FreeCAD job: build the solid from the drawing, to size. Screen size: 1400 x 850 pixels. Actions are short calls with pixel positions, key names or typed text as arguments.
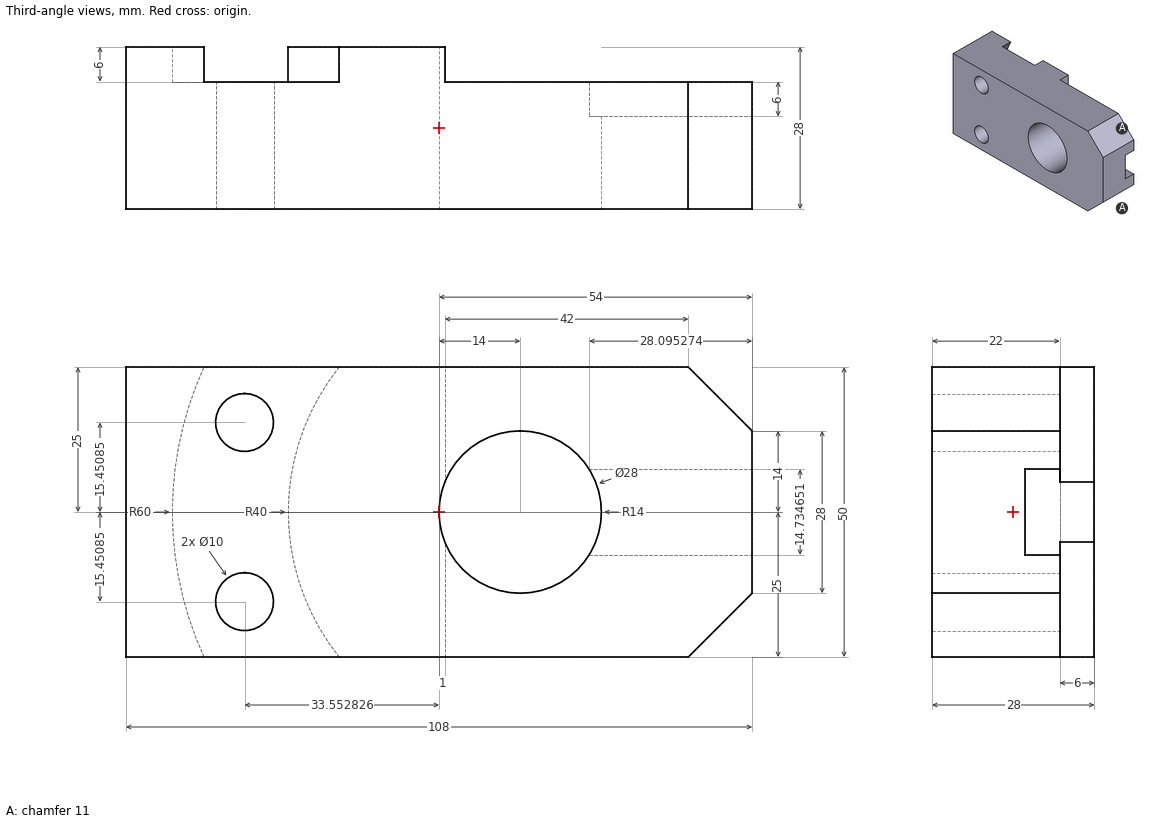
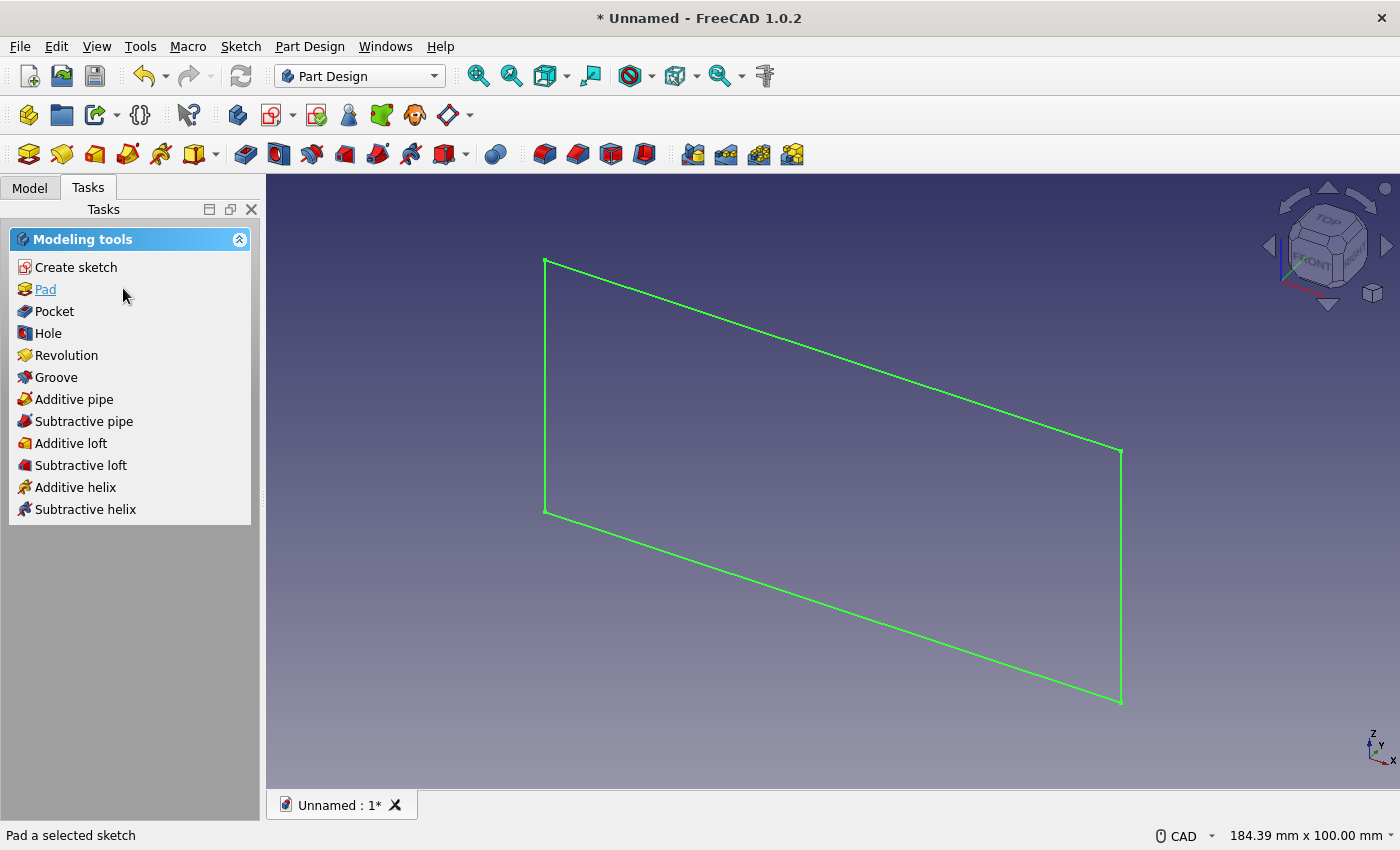
click(29, 154)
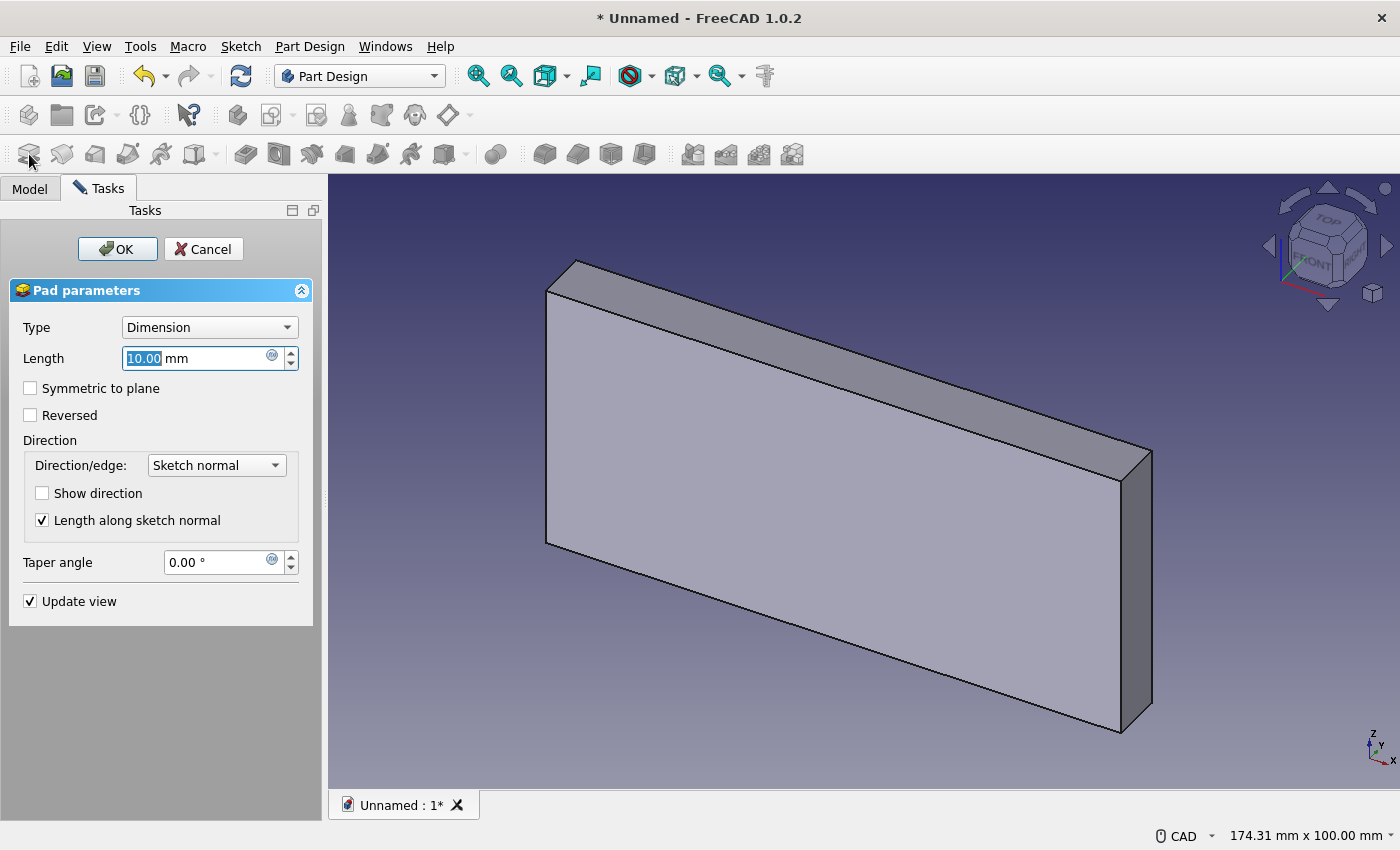
text(28)
key(Tab)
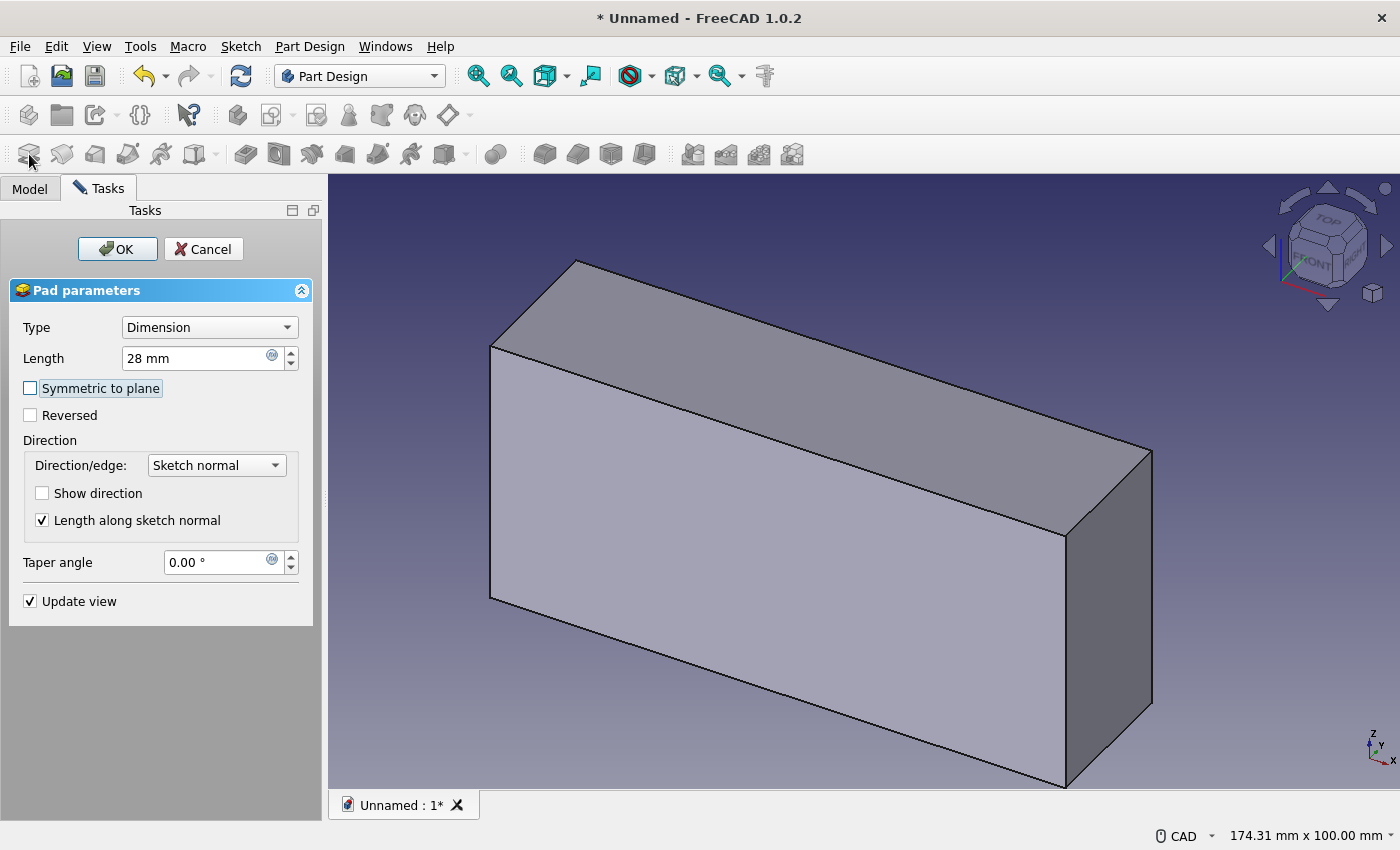
click(31, 388)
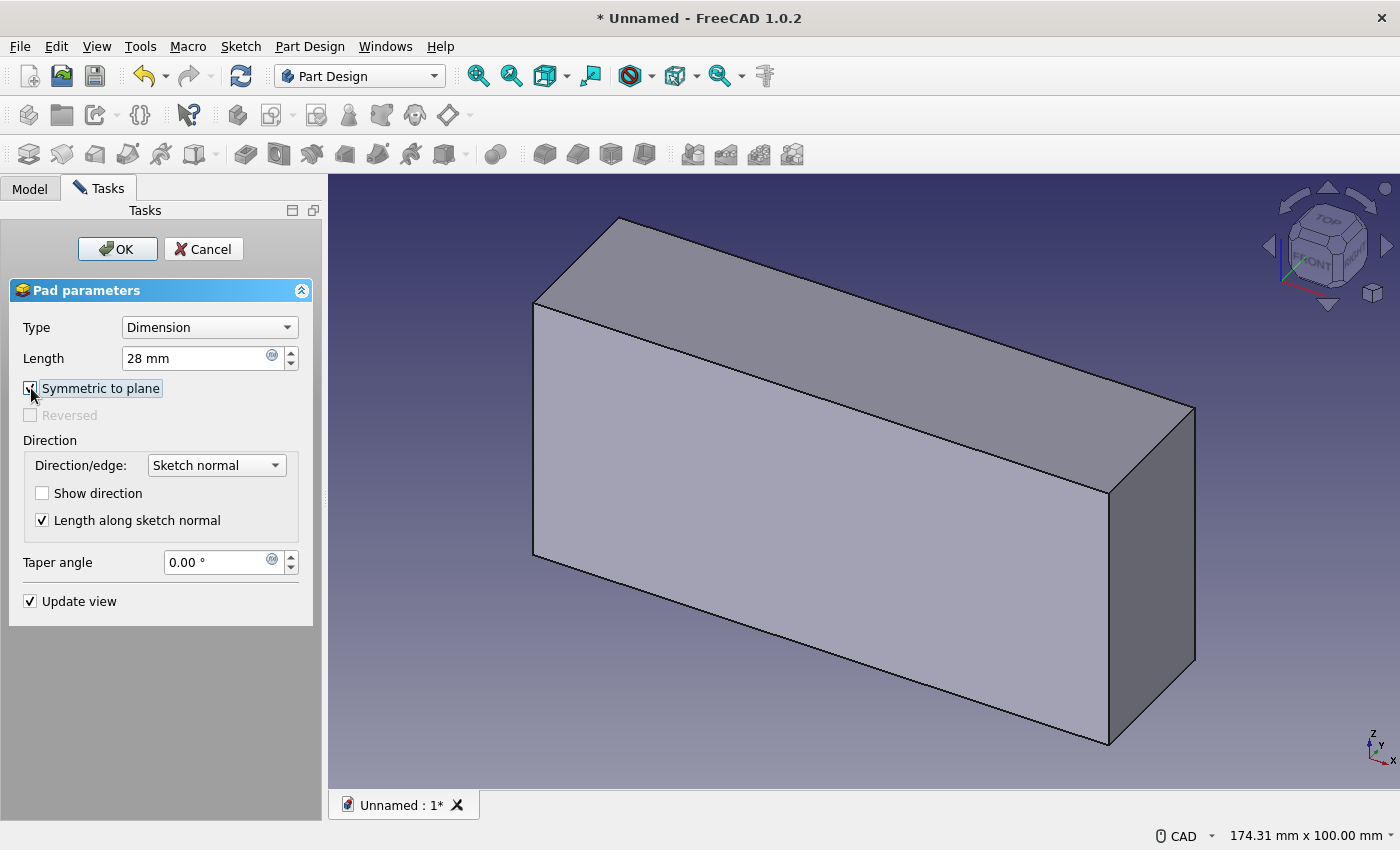
click(118, 249)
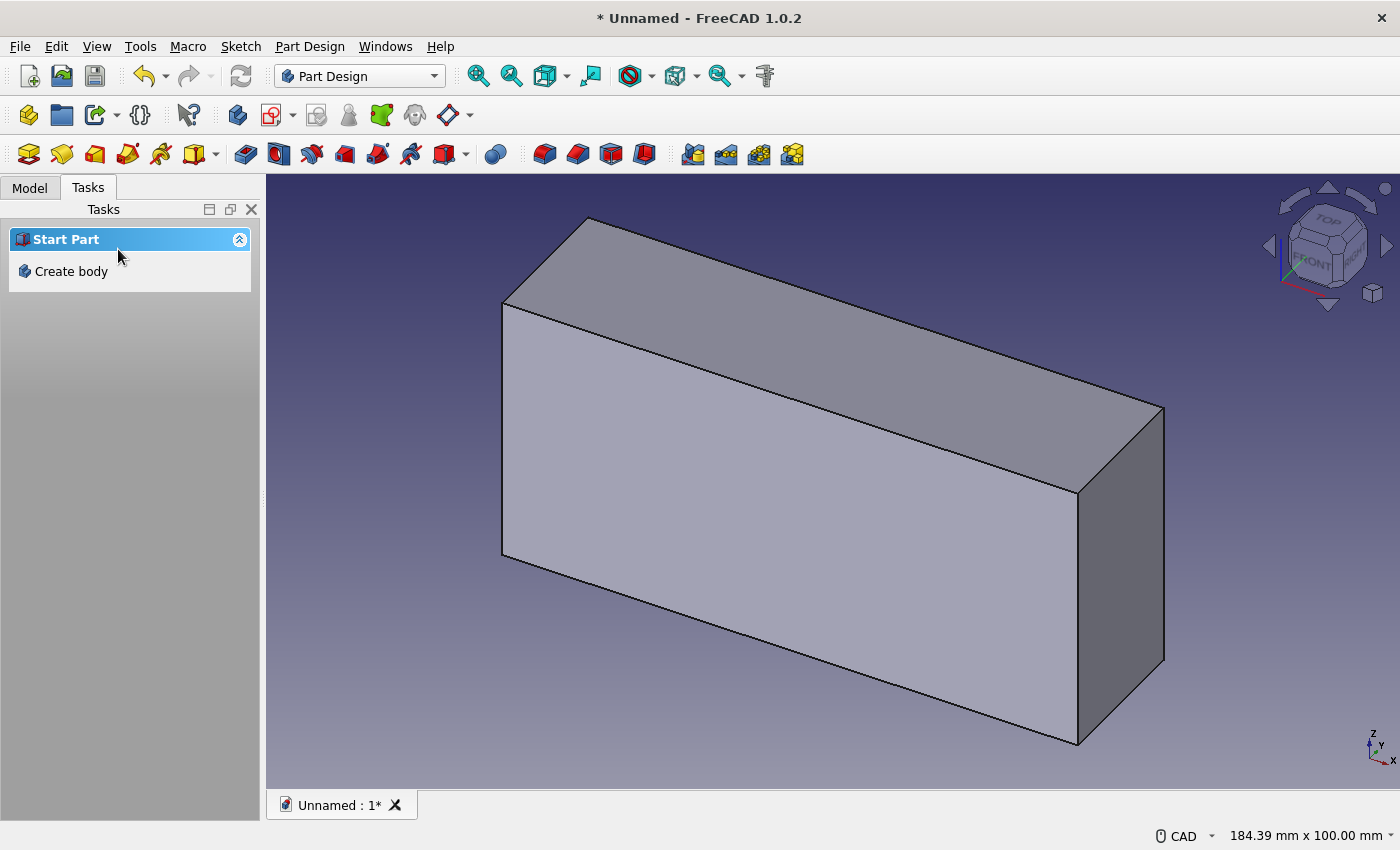
click(1121, 450)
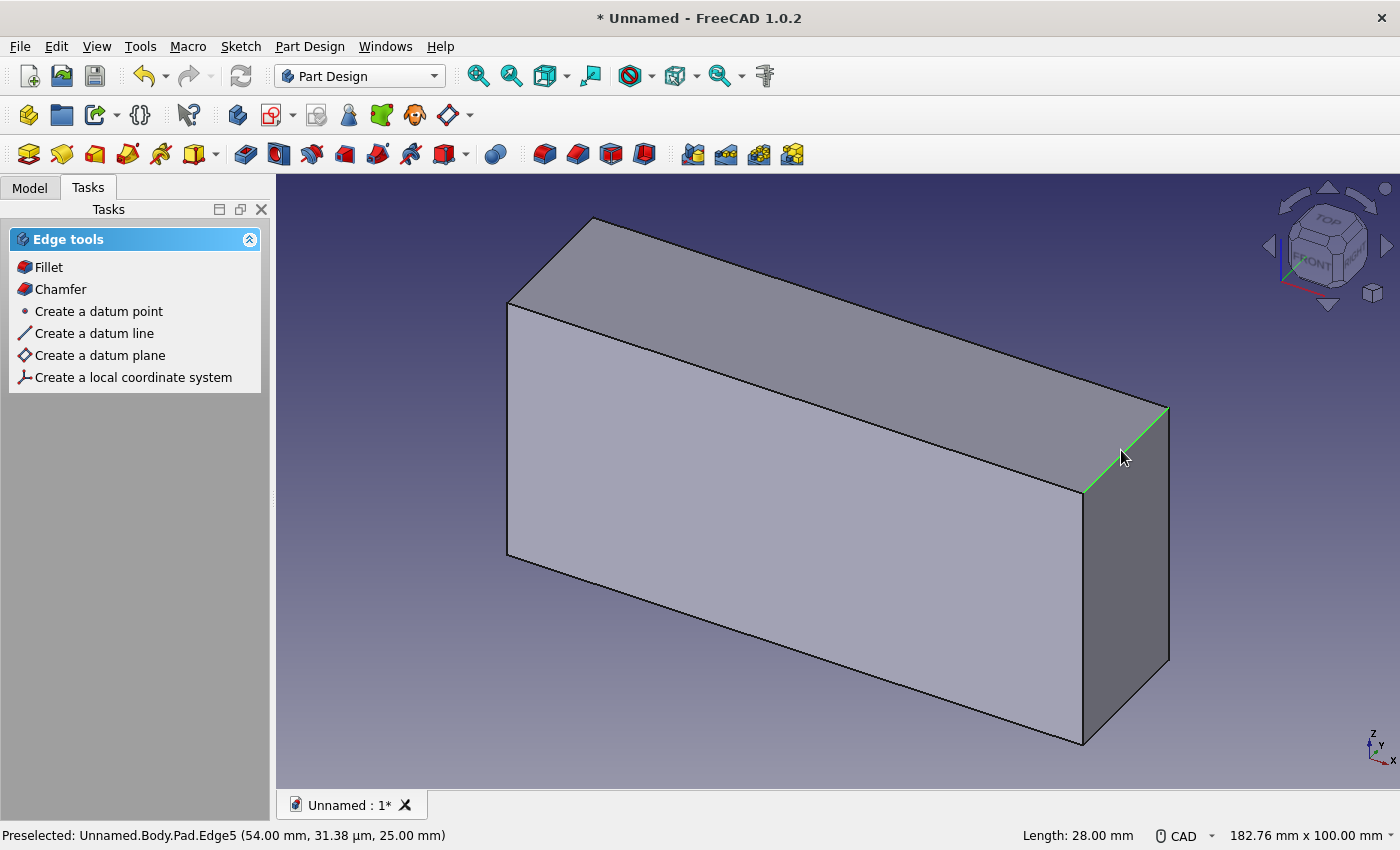
key(0)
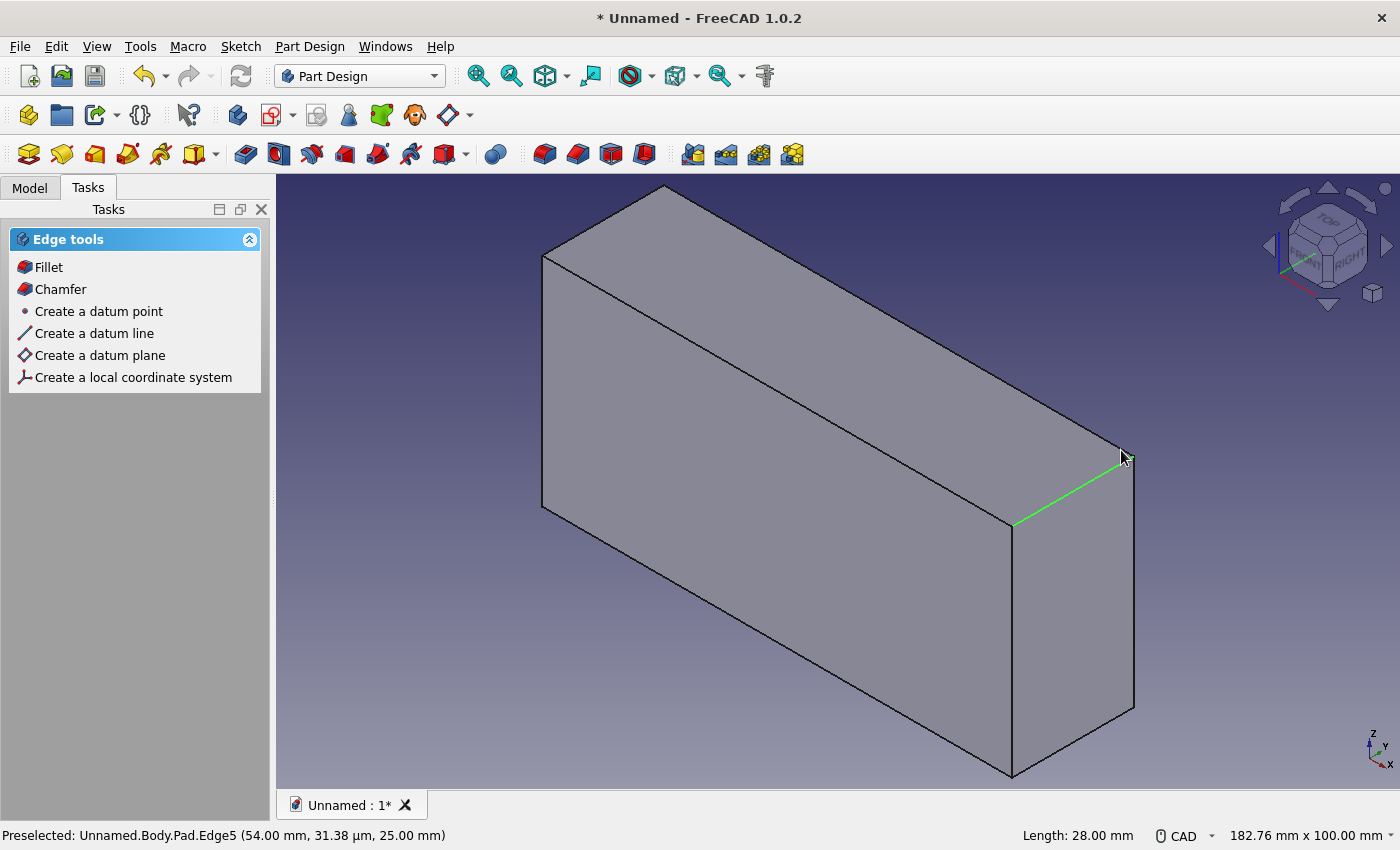
key(2)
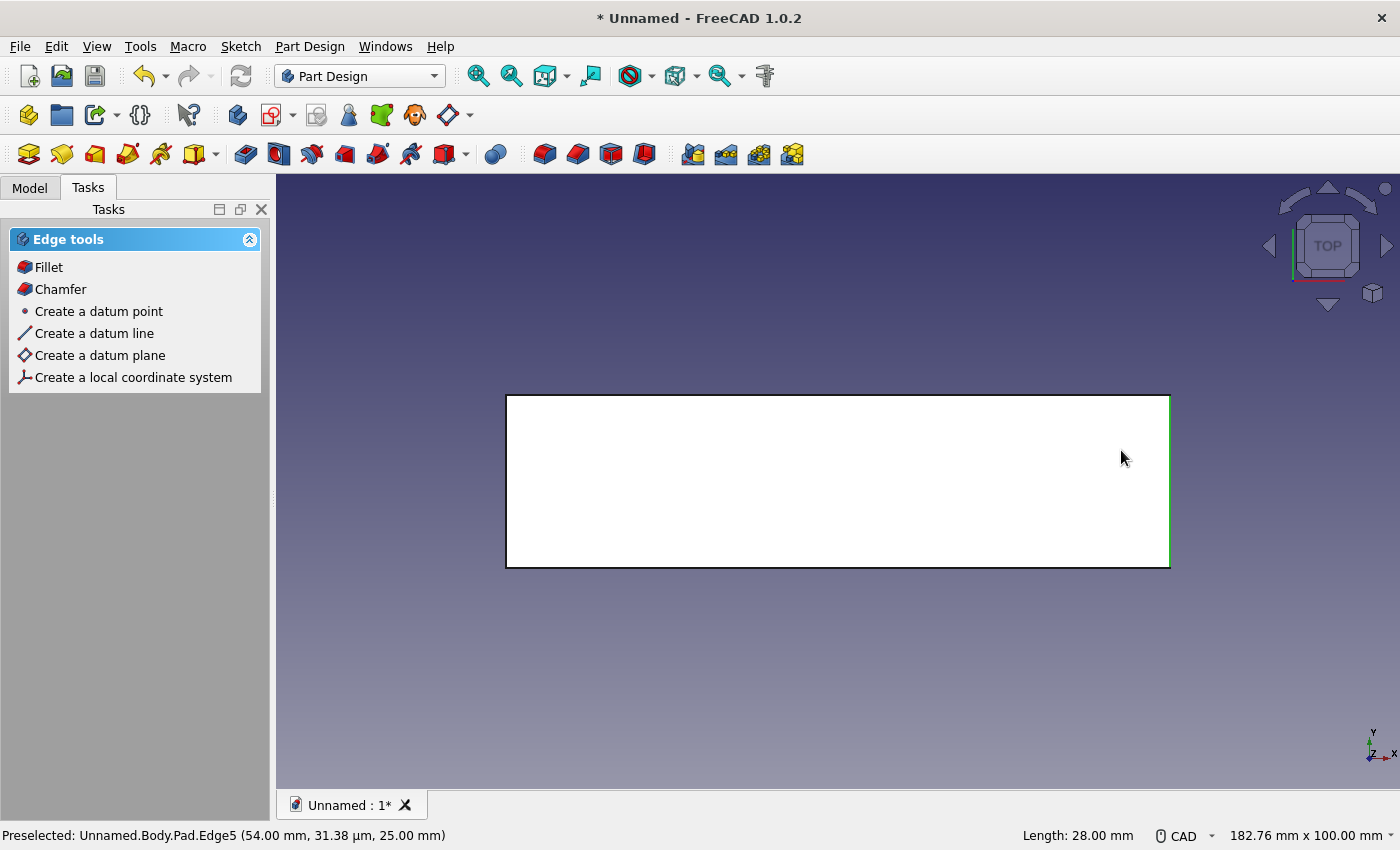
key(1)